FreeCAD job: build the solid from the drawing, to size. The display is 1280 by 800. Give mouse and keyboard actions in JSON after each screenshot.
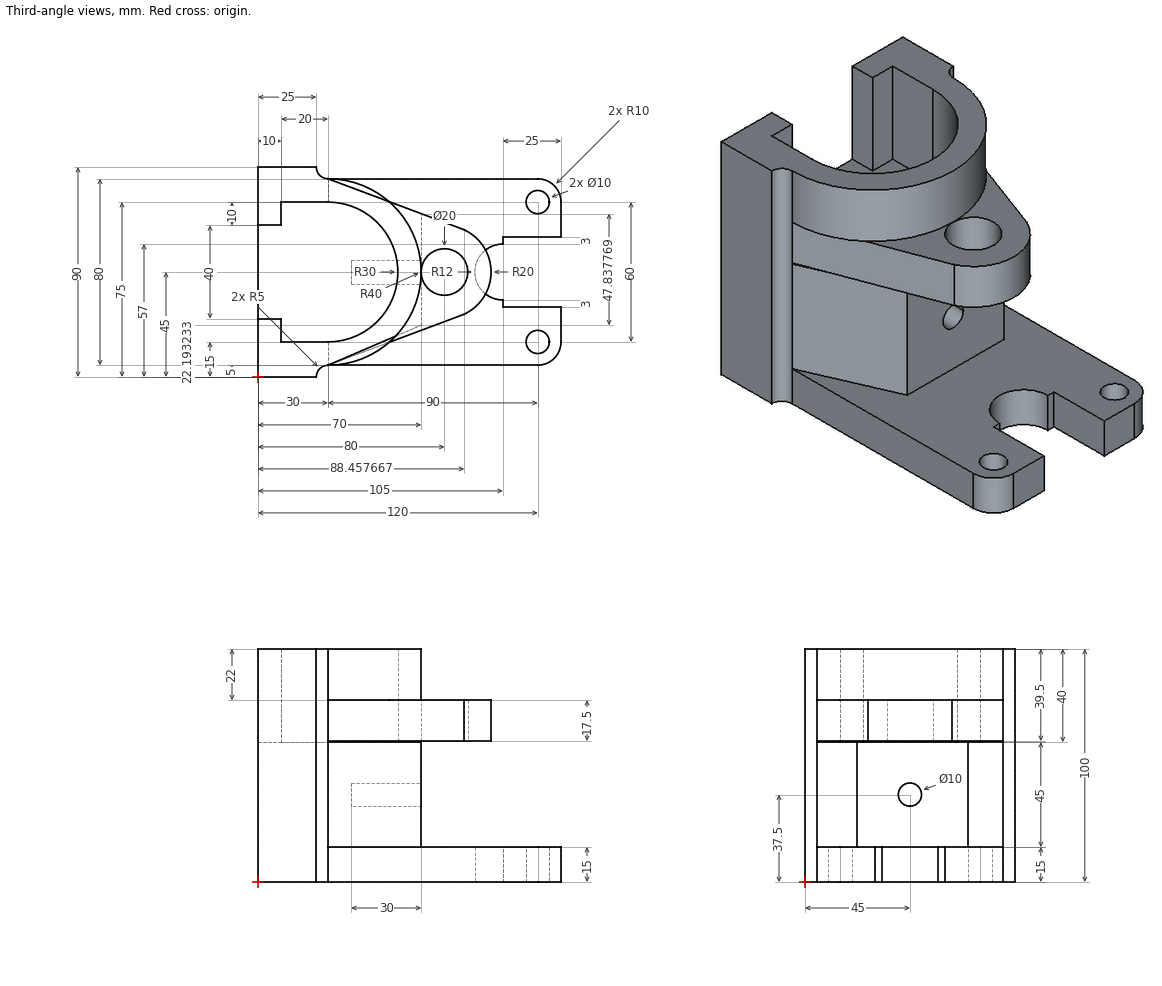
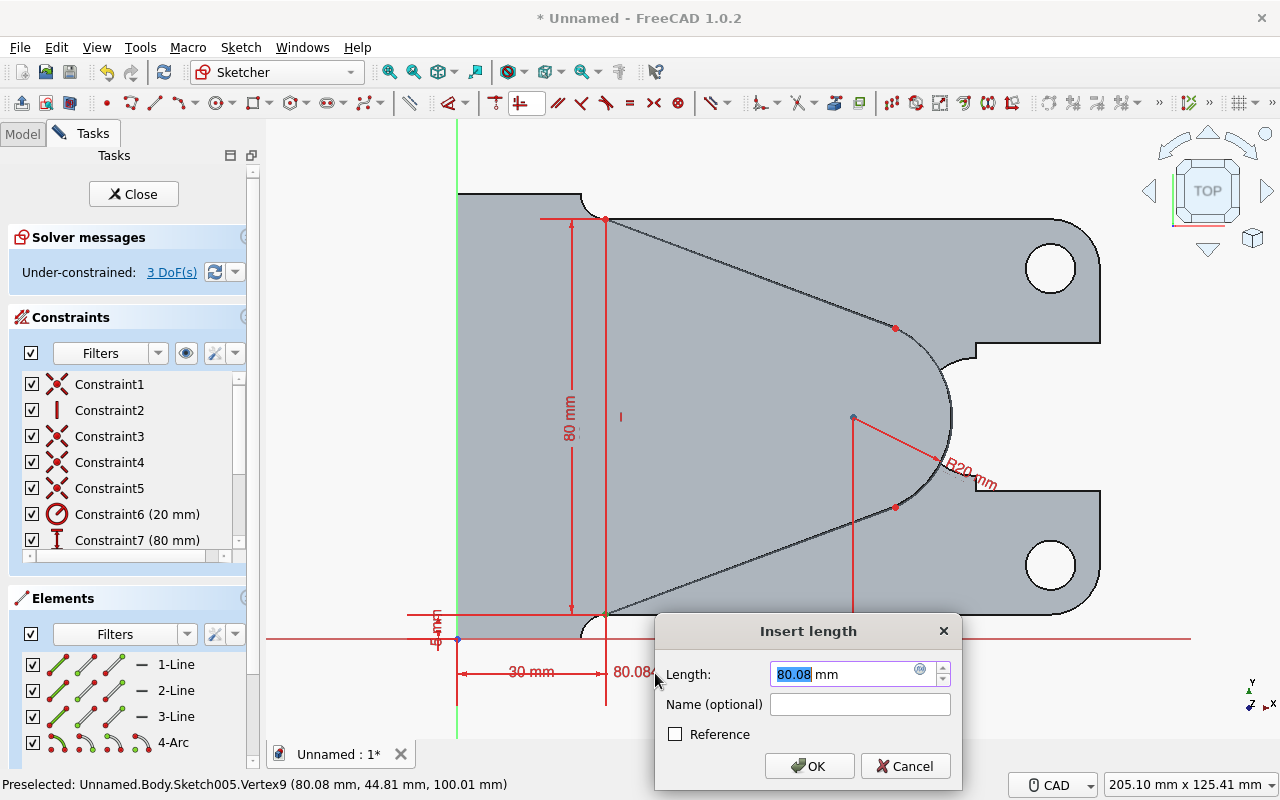
{"action": "type", "text": "80"}
{"action": "key", "text": "Return"}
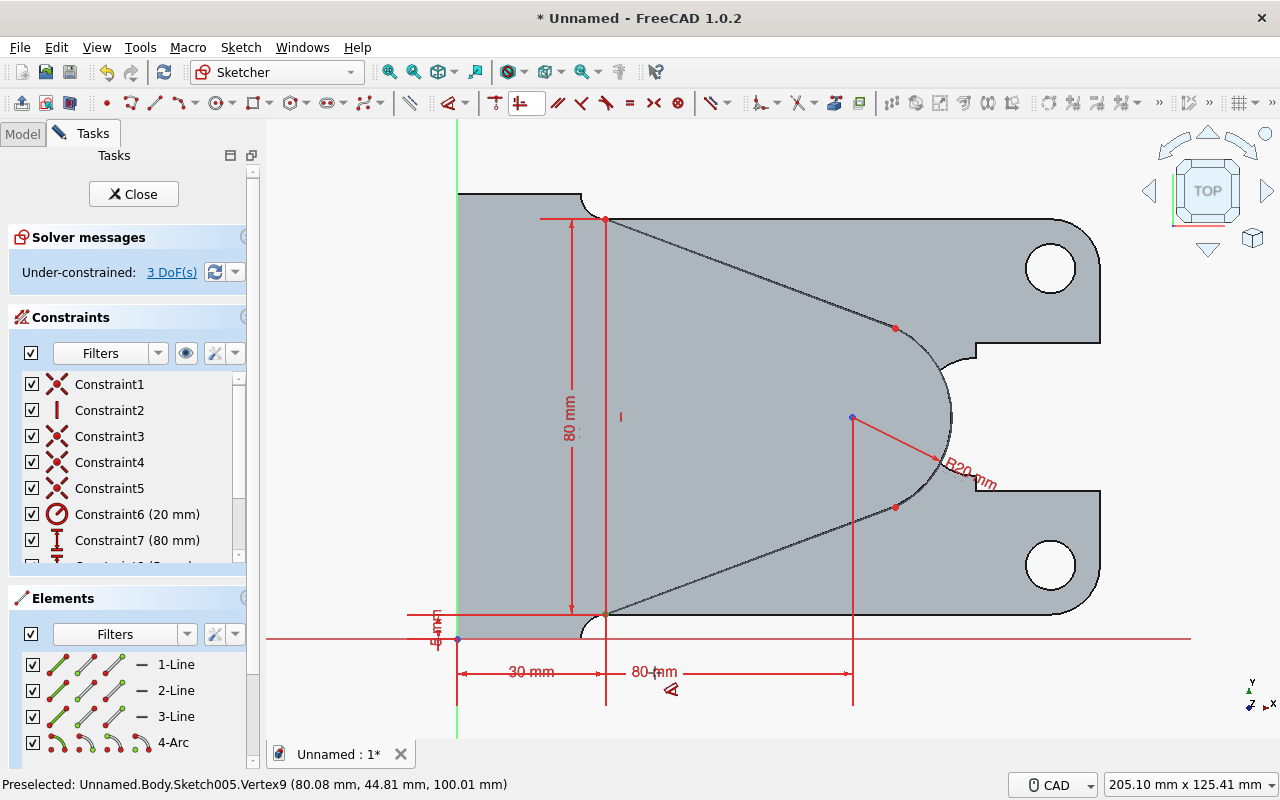
{"action": "left_click", "coordinate": [853, 418]}
{"action": "left_click", "coordinate": [423, 528]}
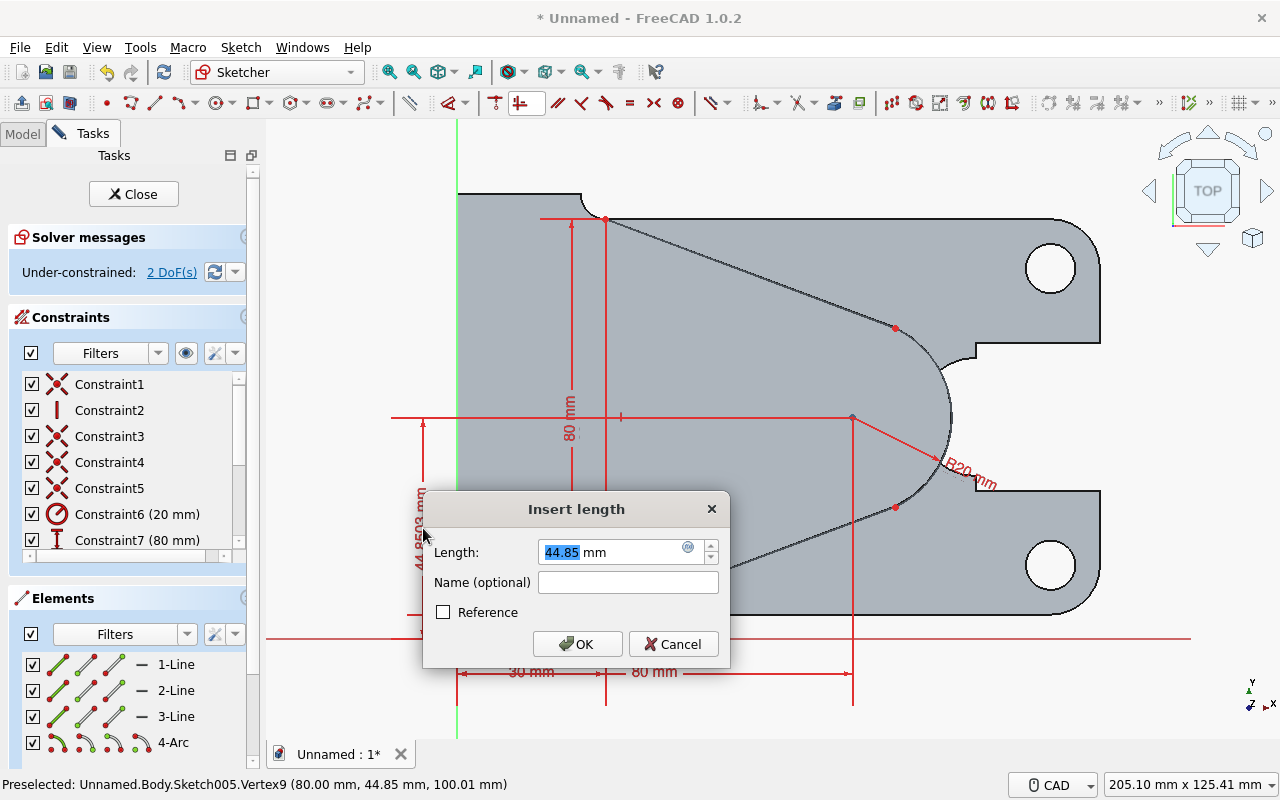
{"action": "type", "text": "45"}
{"action": "key", "text": "Return"}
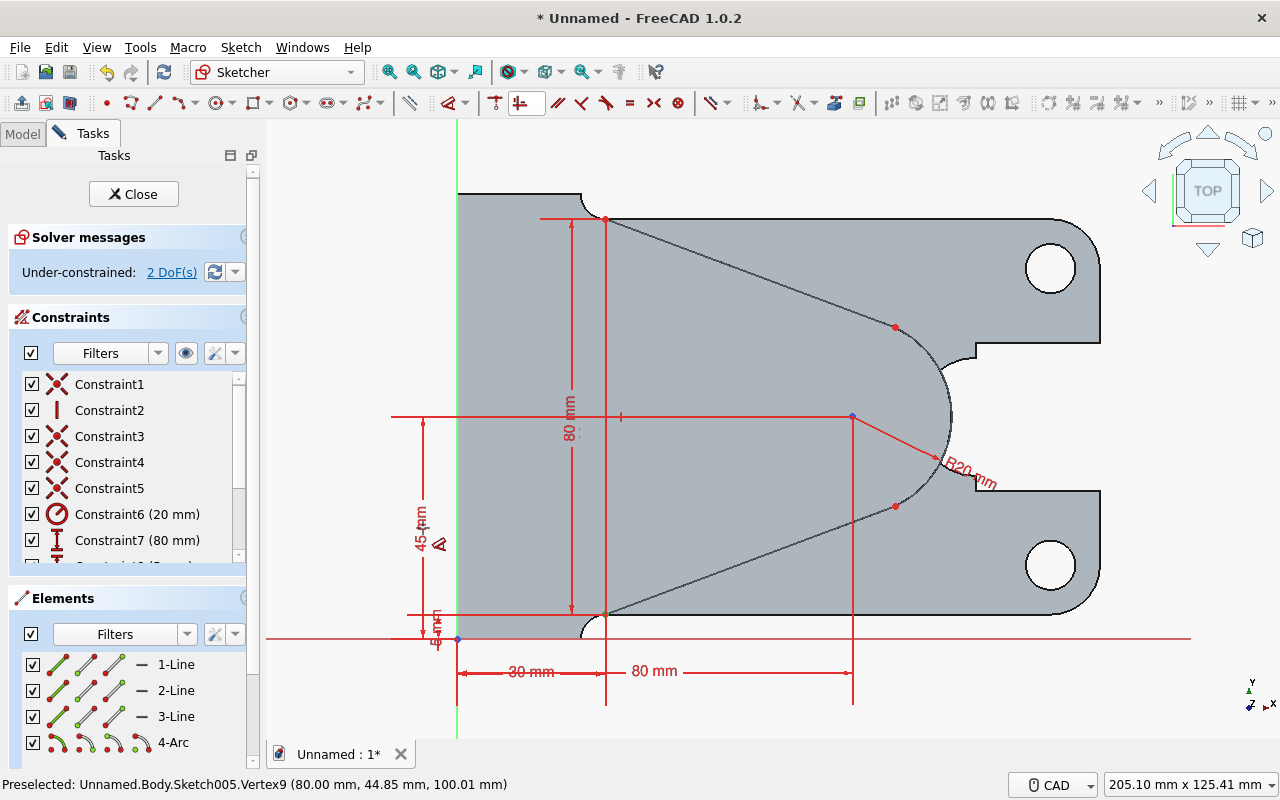
{"action": "left_click", "coordinate": [895, 327]}
{"action": "left_click", "coordinate": [777, 673]}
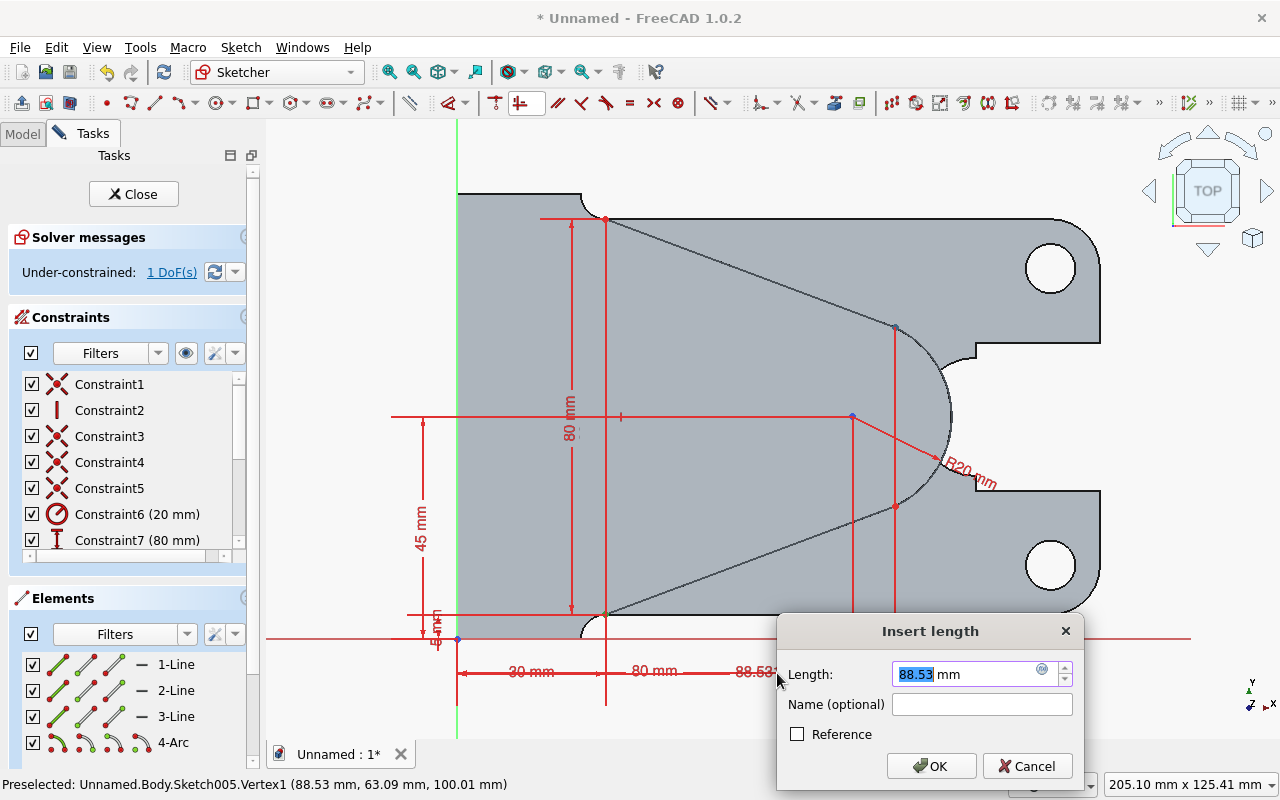
{"action": "type", "text": "88.457667"}
{"action": "key", "text": "Return"}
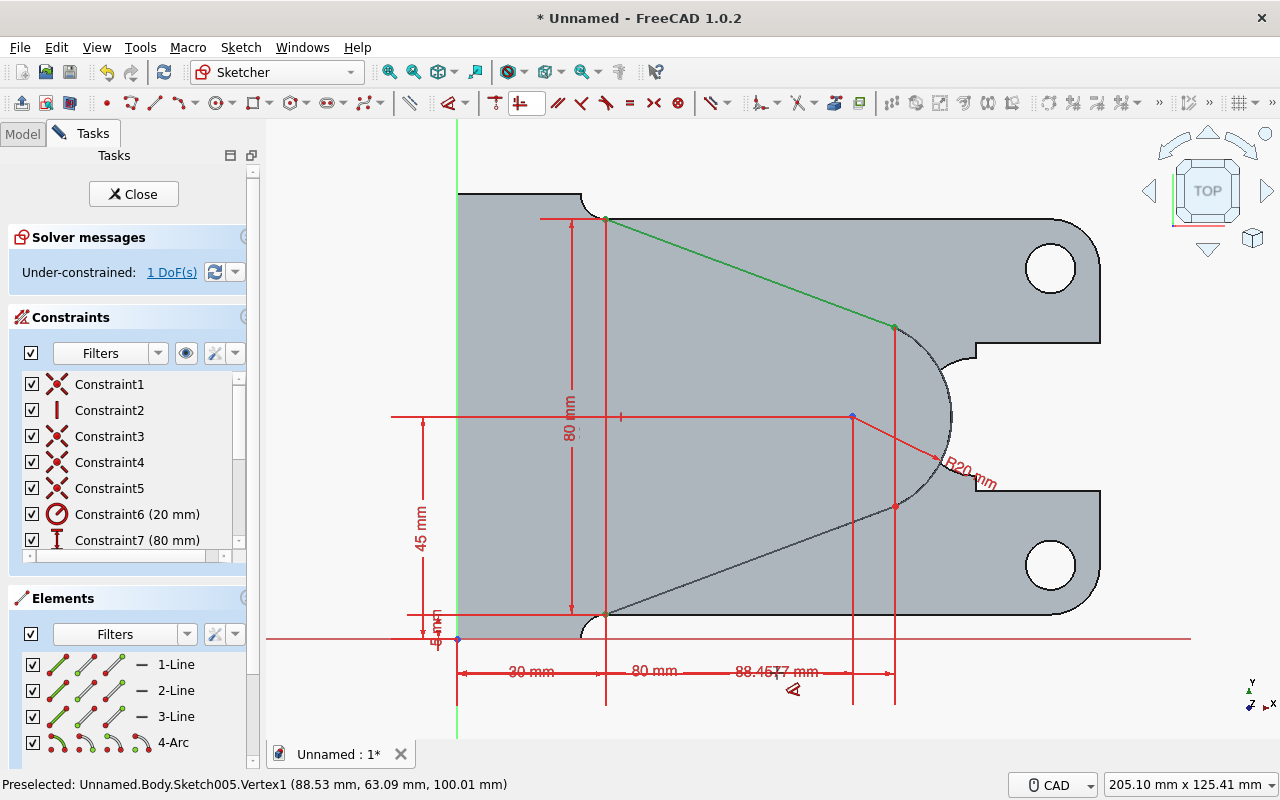
{"action": "left_click", "coordinate": [895, 506]}
{"action": "left_click", "coordinate": [676, 472]}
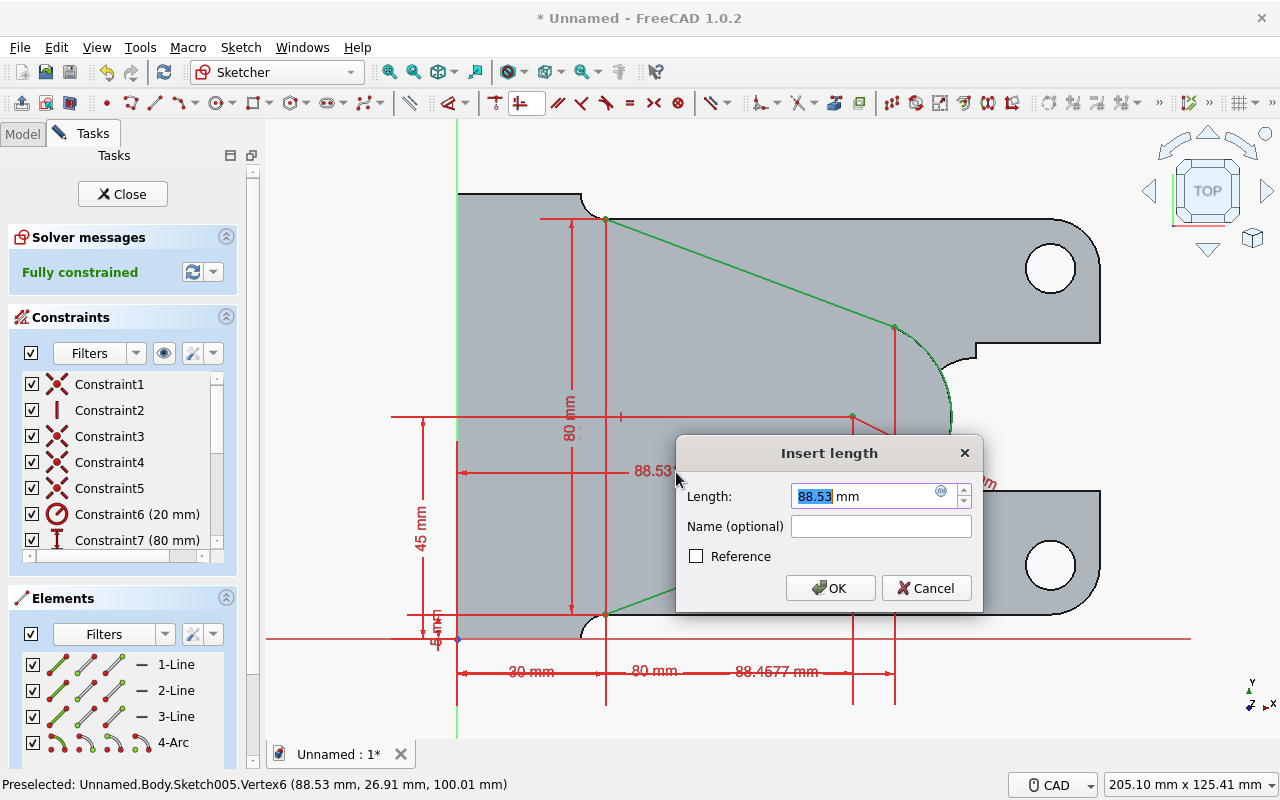
{"action": "type", "text": "88.457667"}
{"action": "key", "text": "Return"}
{"action": "key", "text": "Escape"}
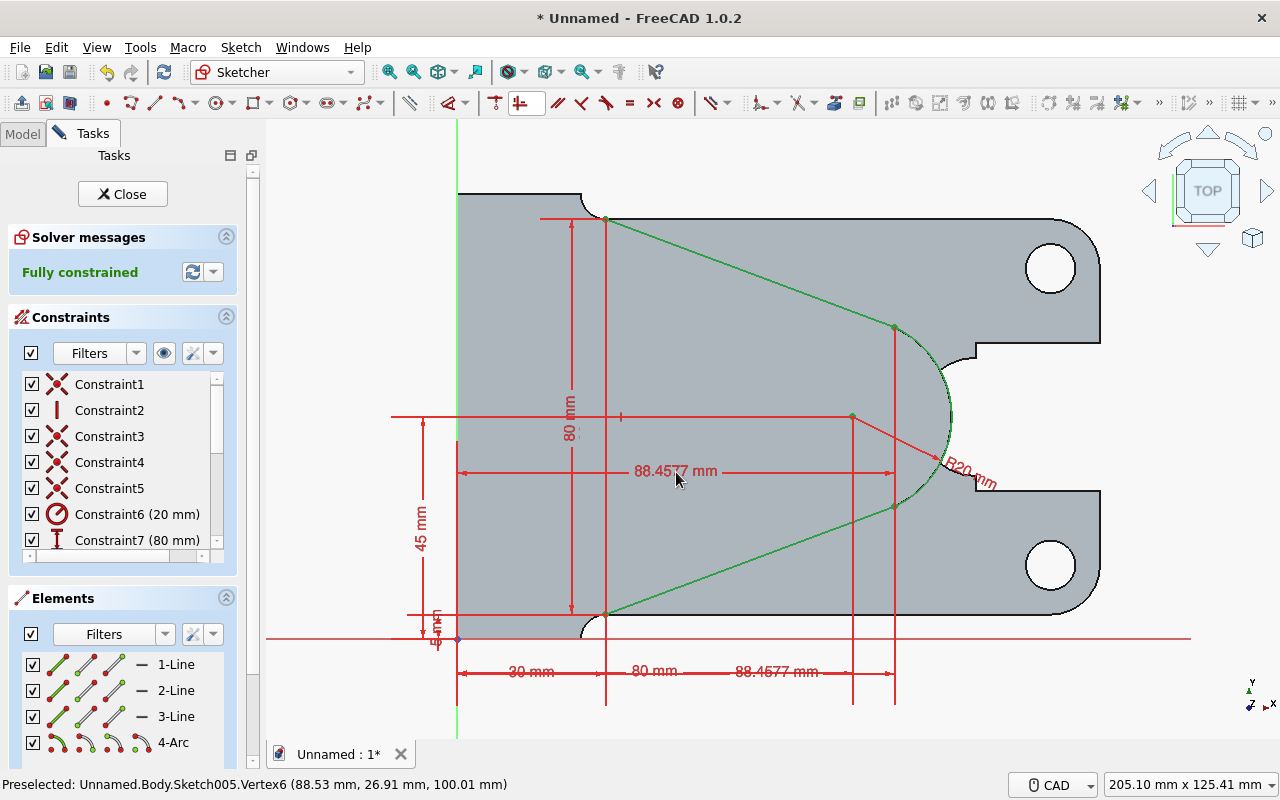
{"action": "left_click", "coordinate": [123, 194]}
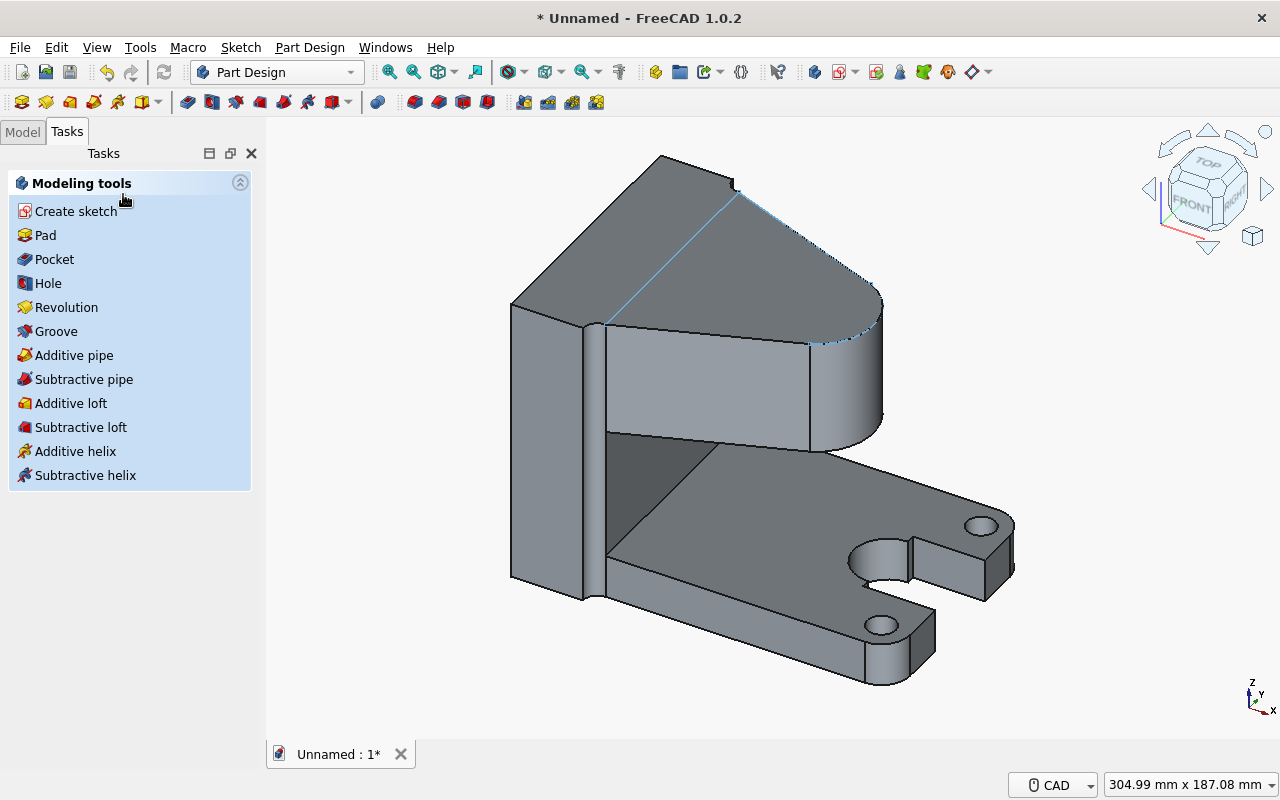
{"action": "left_click", "coordinate": [188, 102]}